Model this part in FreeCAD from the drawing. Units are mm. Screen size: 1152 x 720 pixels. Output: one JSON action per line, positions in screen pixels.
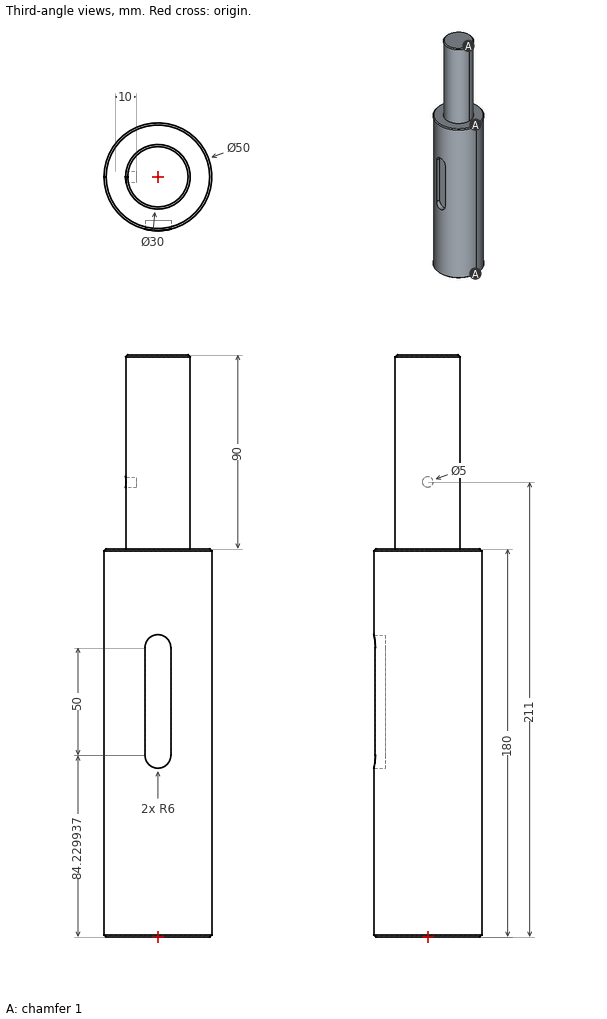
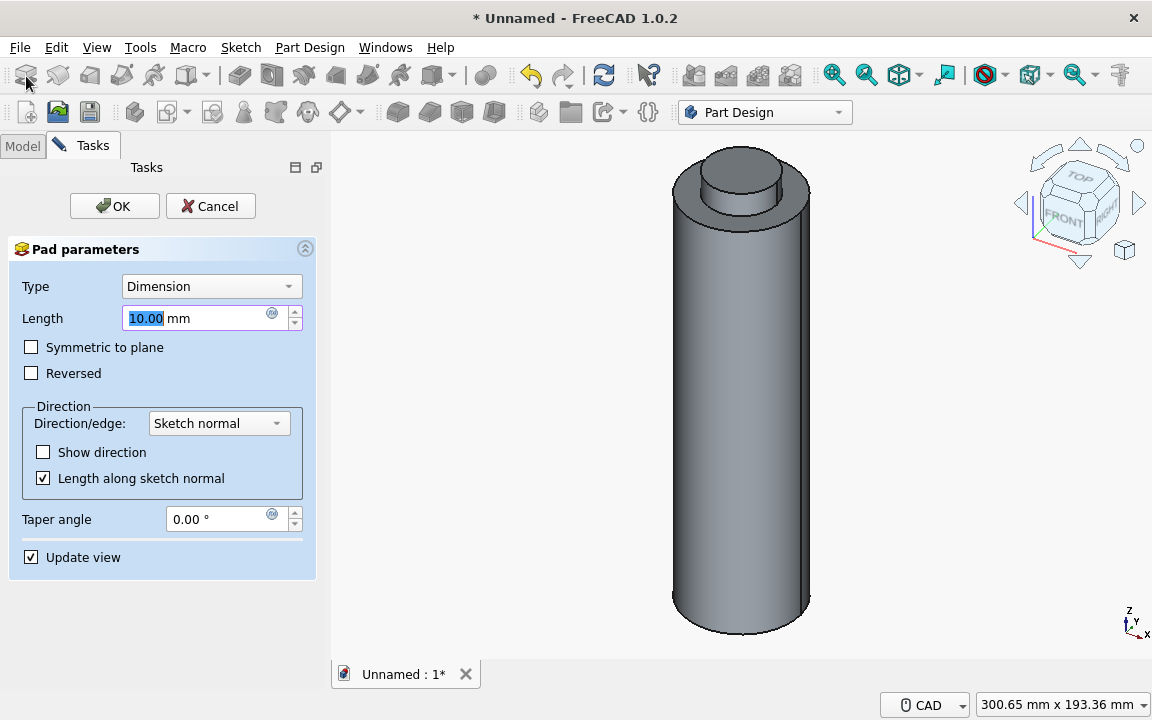
{"action": "type", "text": "90"}
{"action": "key", "text": "Tab"}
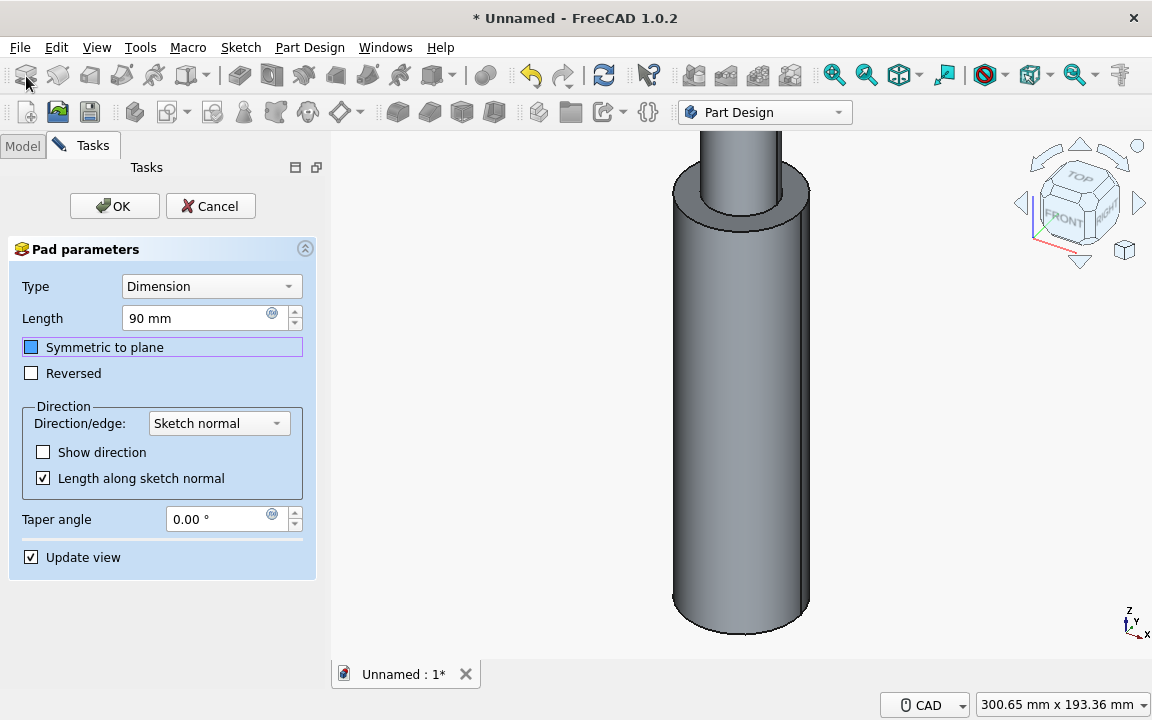
{"action": "left_click", "coordinate": [115, 206]}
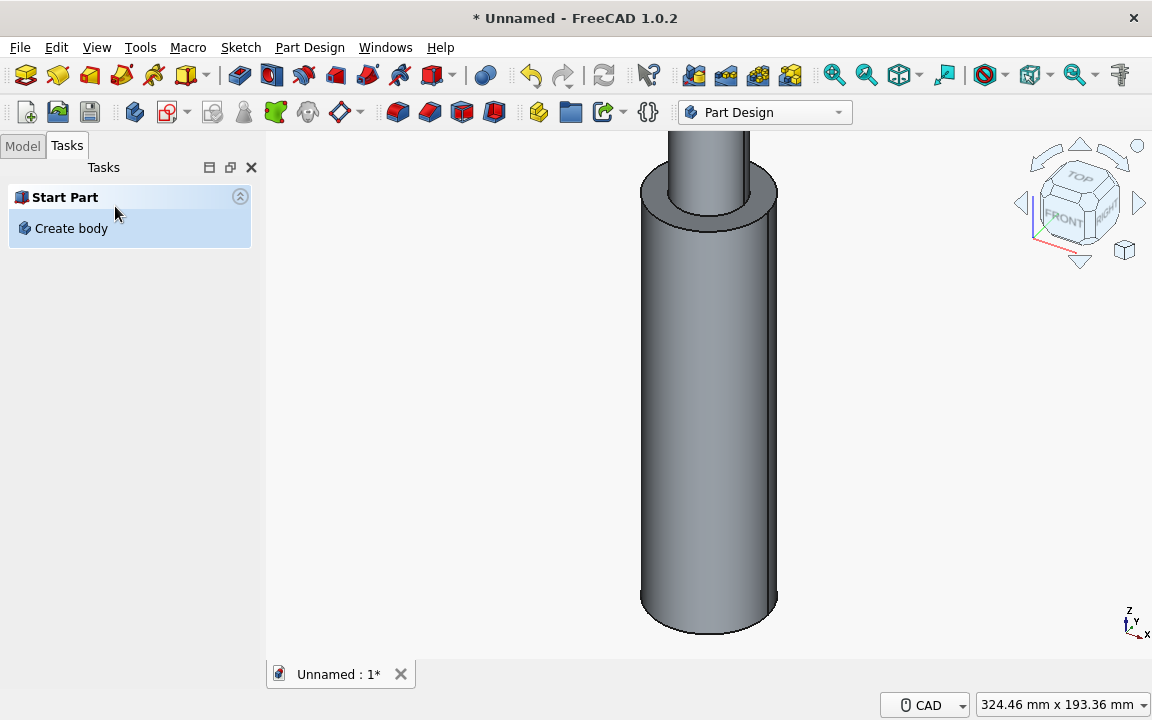
{"action": "key", "text": "v f"}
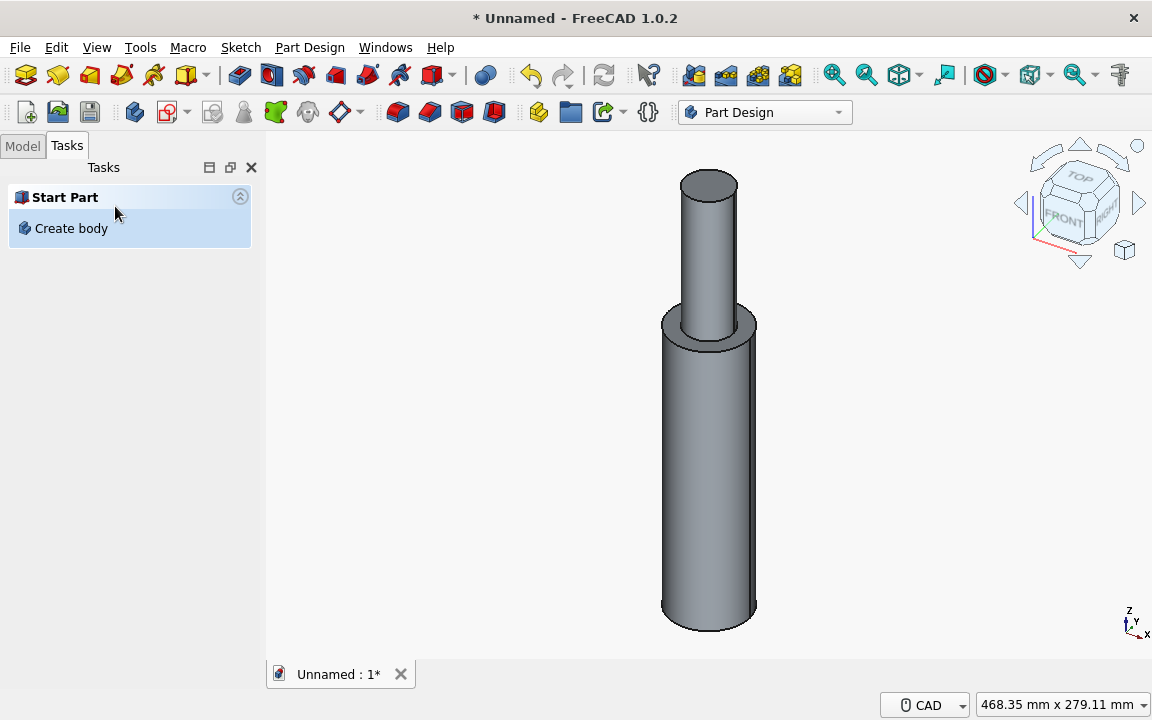
{"action": "left_click", "coordinate": [23, 145]}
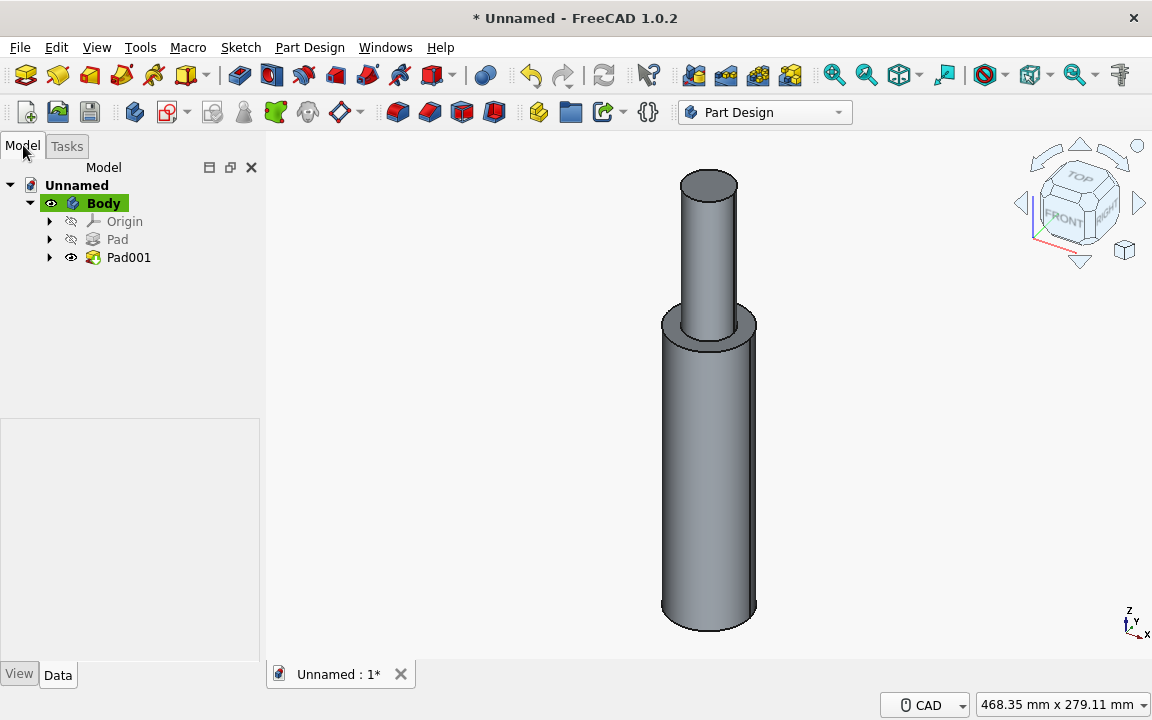
{"action": "left_click", "coordinate": [50, 221]}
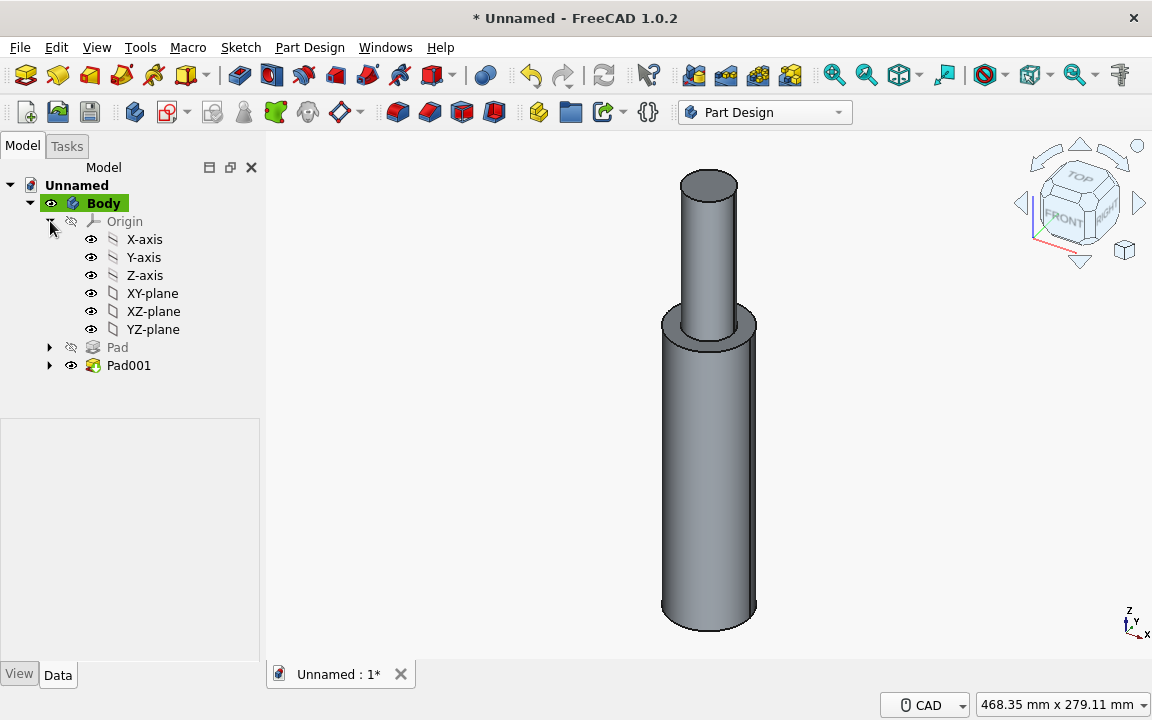
{"action": "left_click", "coordinate": [136, 311]}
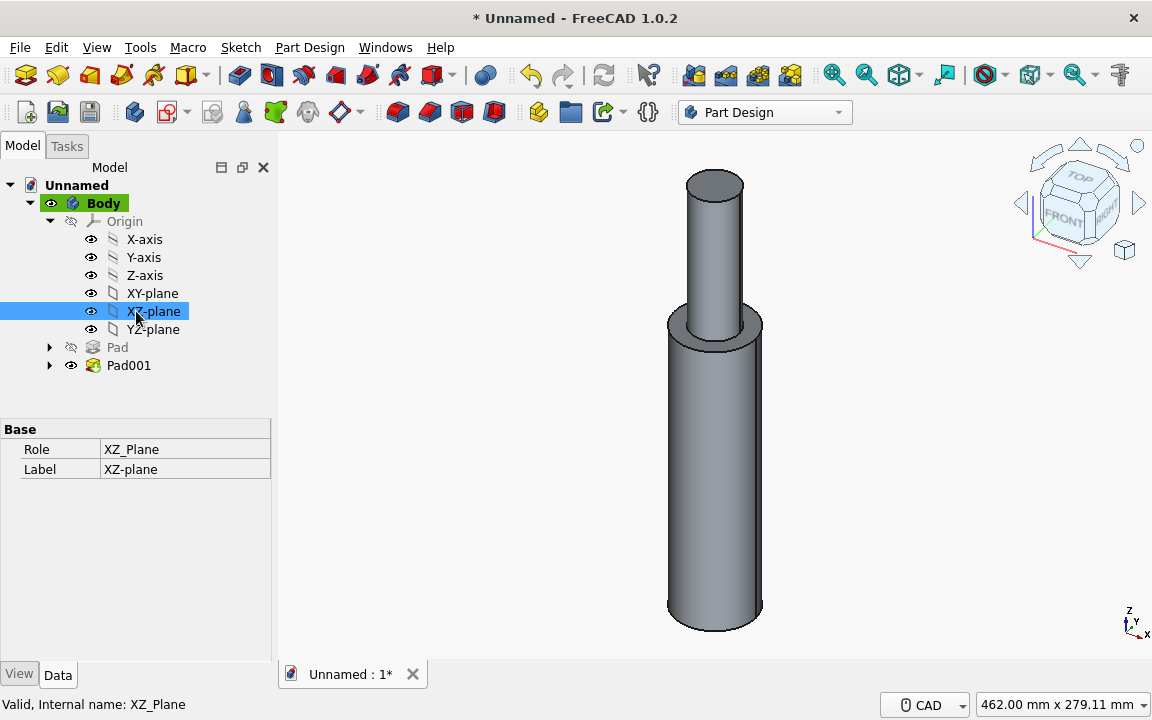
{"action": "left_click", "coordinate": [340, 112]}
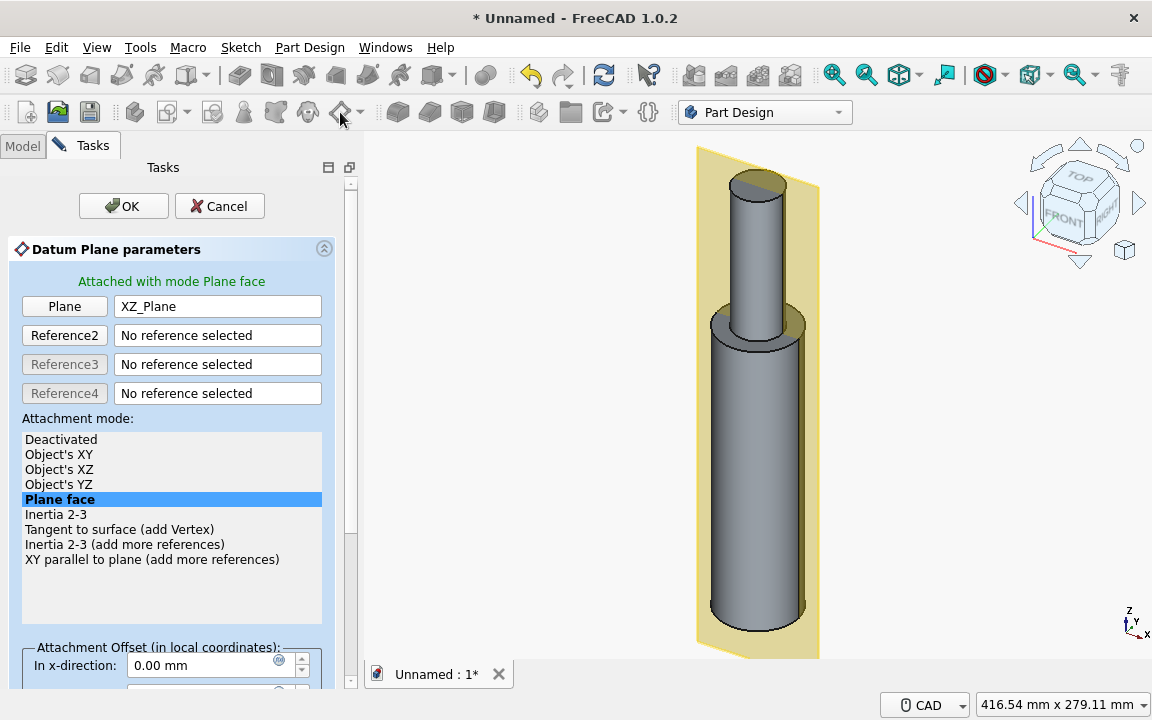
{"action": "scroll", "coordinate": [351, 432], "scroll_direction": "down", "scroll_amount": 2}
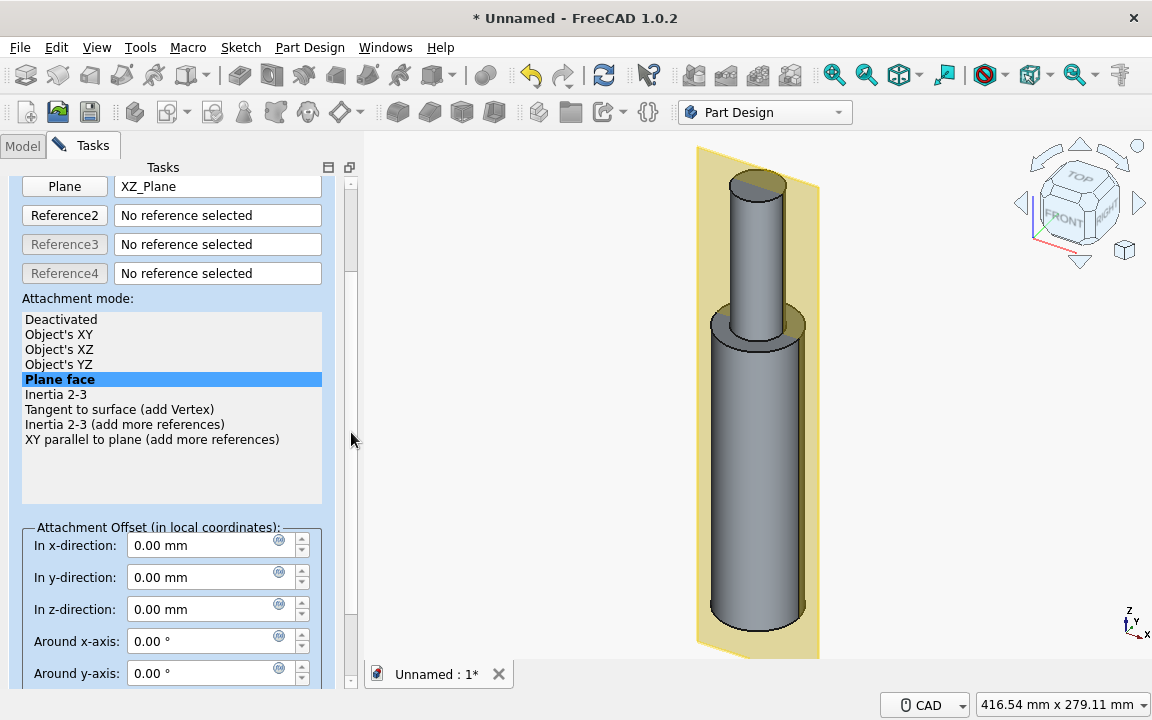
{"action": "triple_click", "coordinate": [210, 609]}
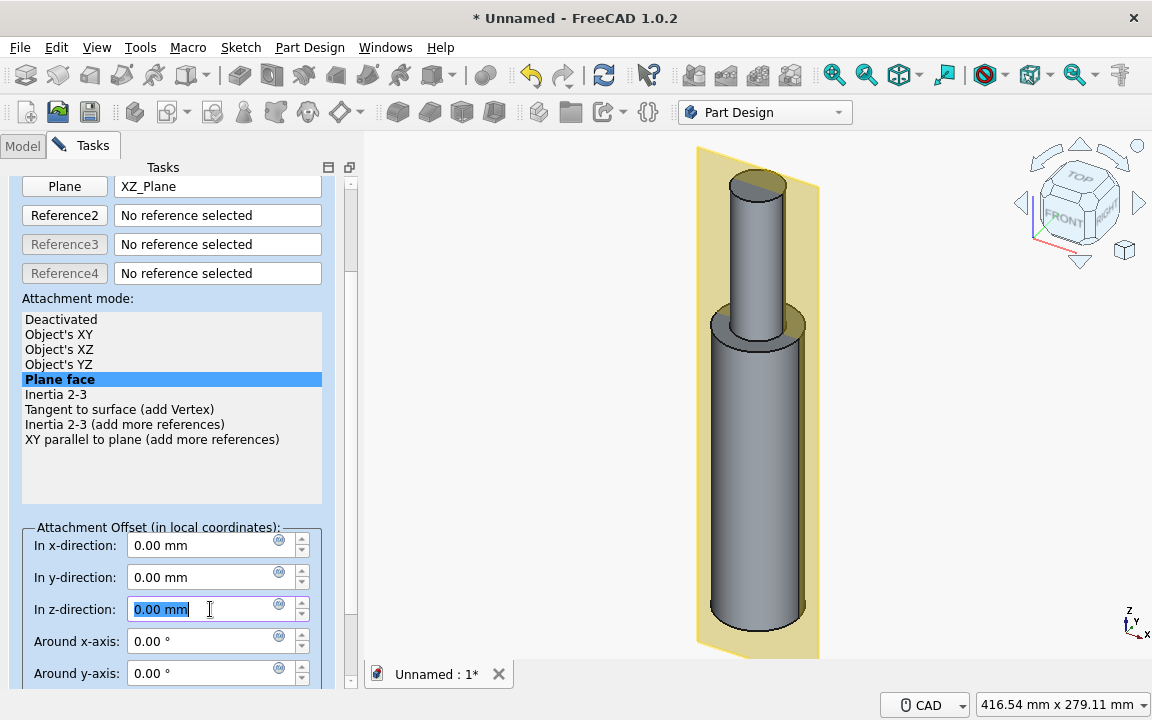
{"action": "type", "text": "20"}
{"action": "key", "text": "Tab"}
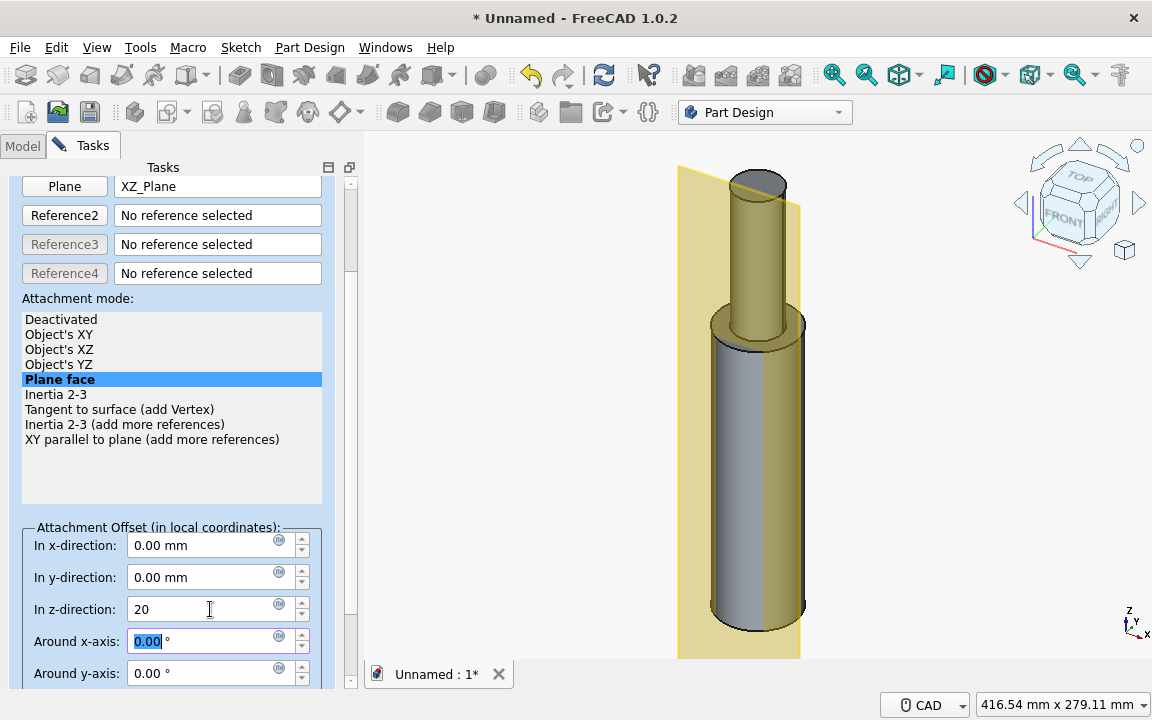
{"action": "scroll", "coordinate": [351, 432], "scroll_direction": "up", "scroll_amount": 3}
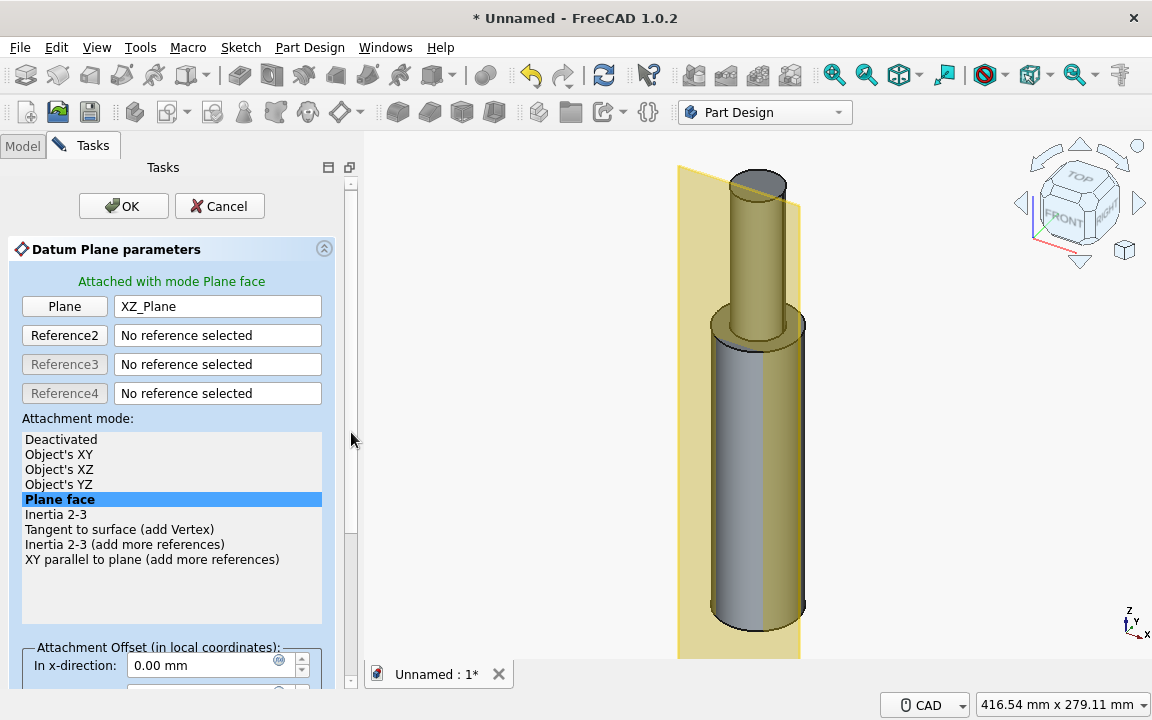
{"action": "left_click", "coordinate": [124, 206]}